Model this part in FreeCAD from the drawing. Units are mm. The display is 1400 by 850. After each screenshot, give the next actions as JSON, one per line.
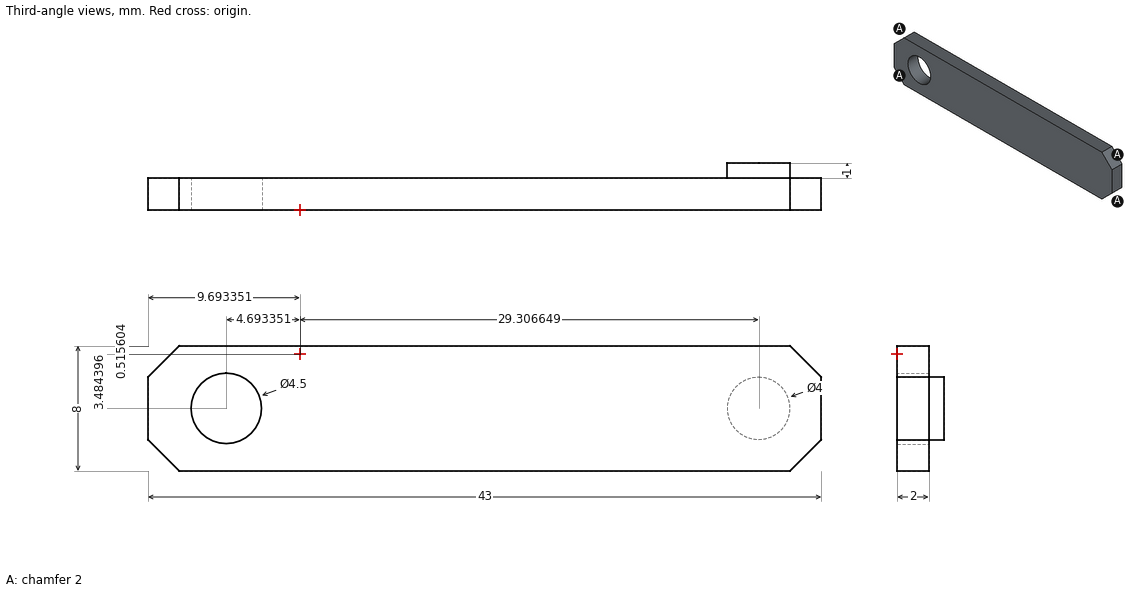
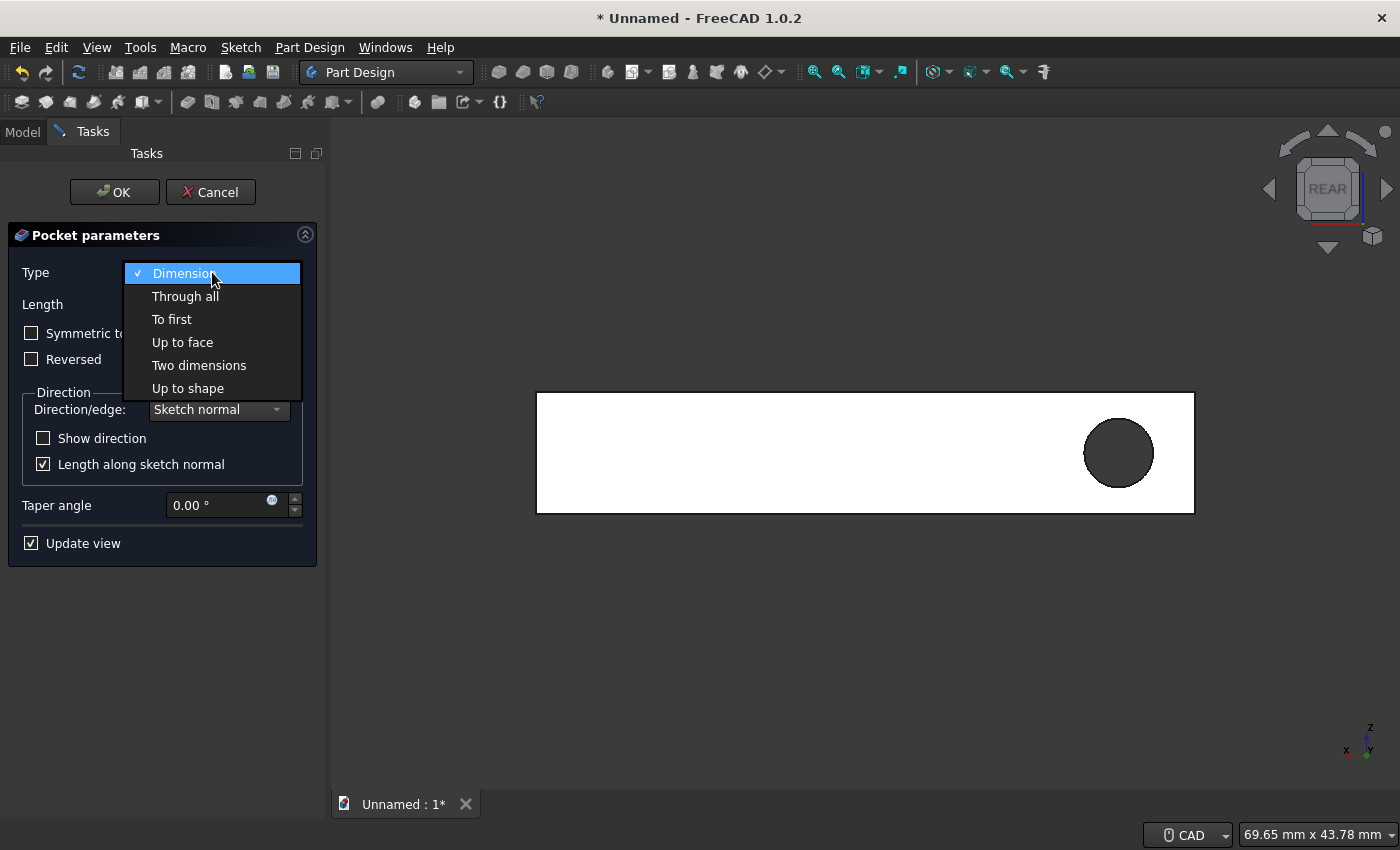
{"action": "left_click", "coordinate": [212, 296]}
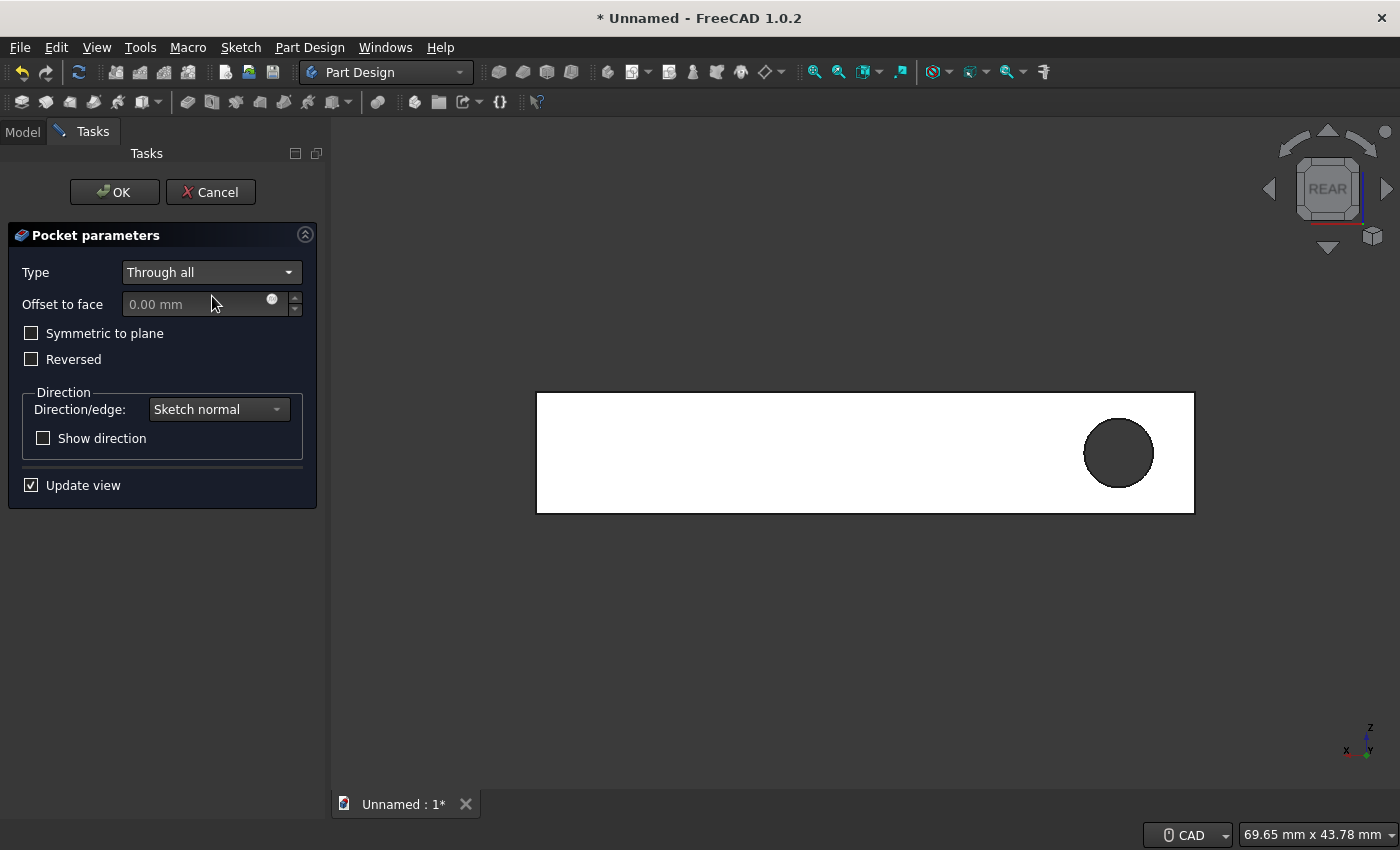
{"action": "left_click", "coordinate": [115, 192]}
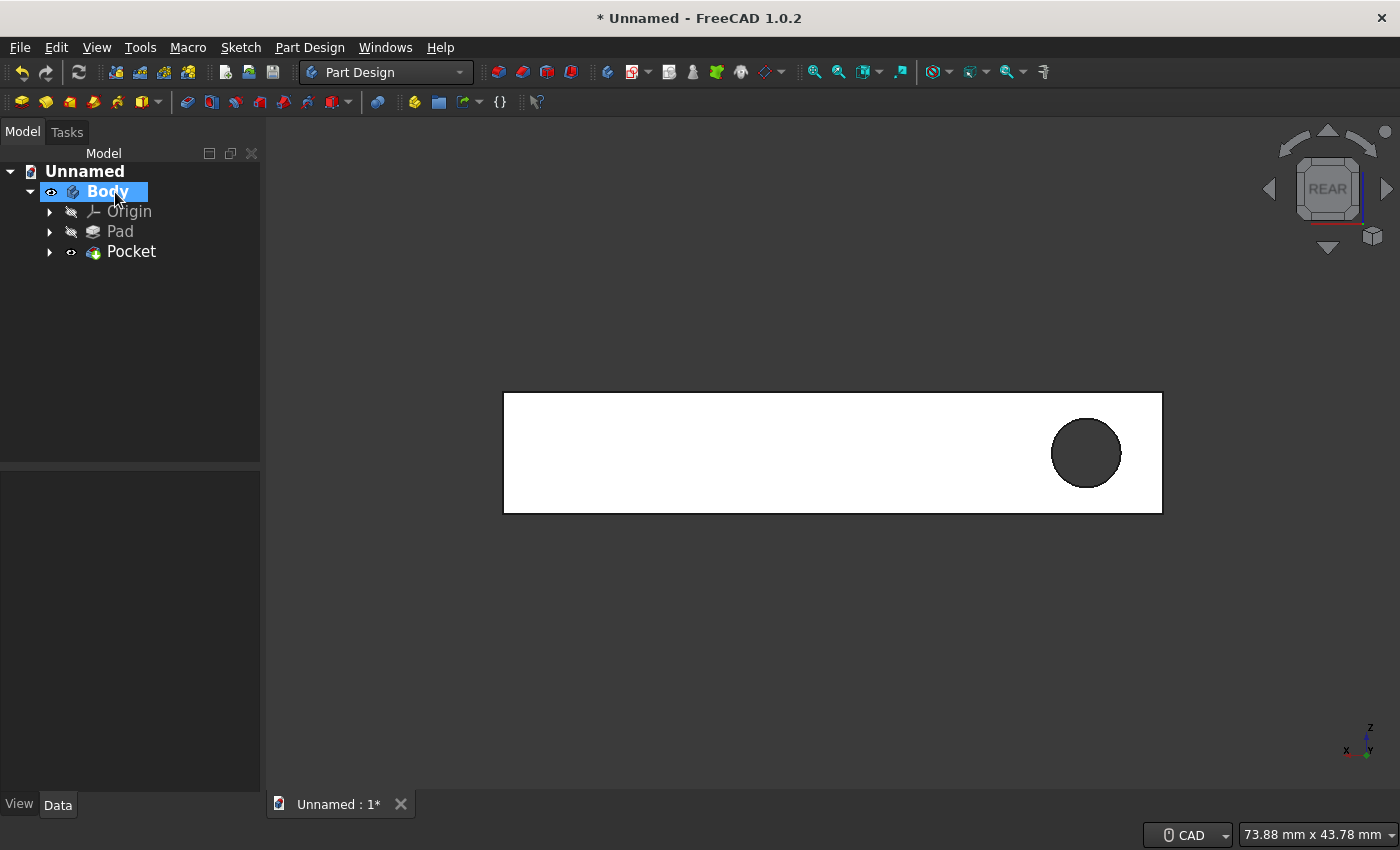
{"action": "left_click", "coordinate": [644, 452]}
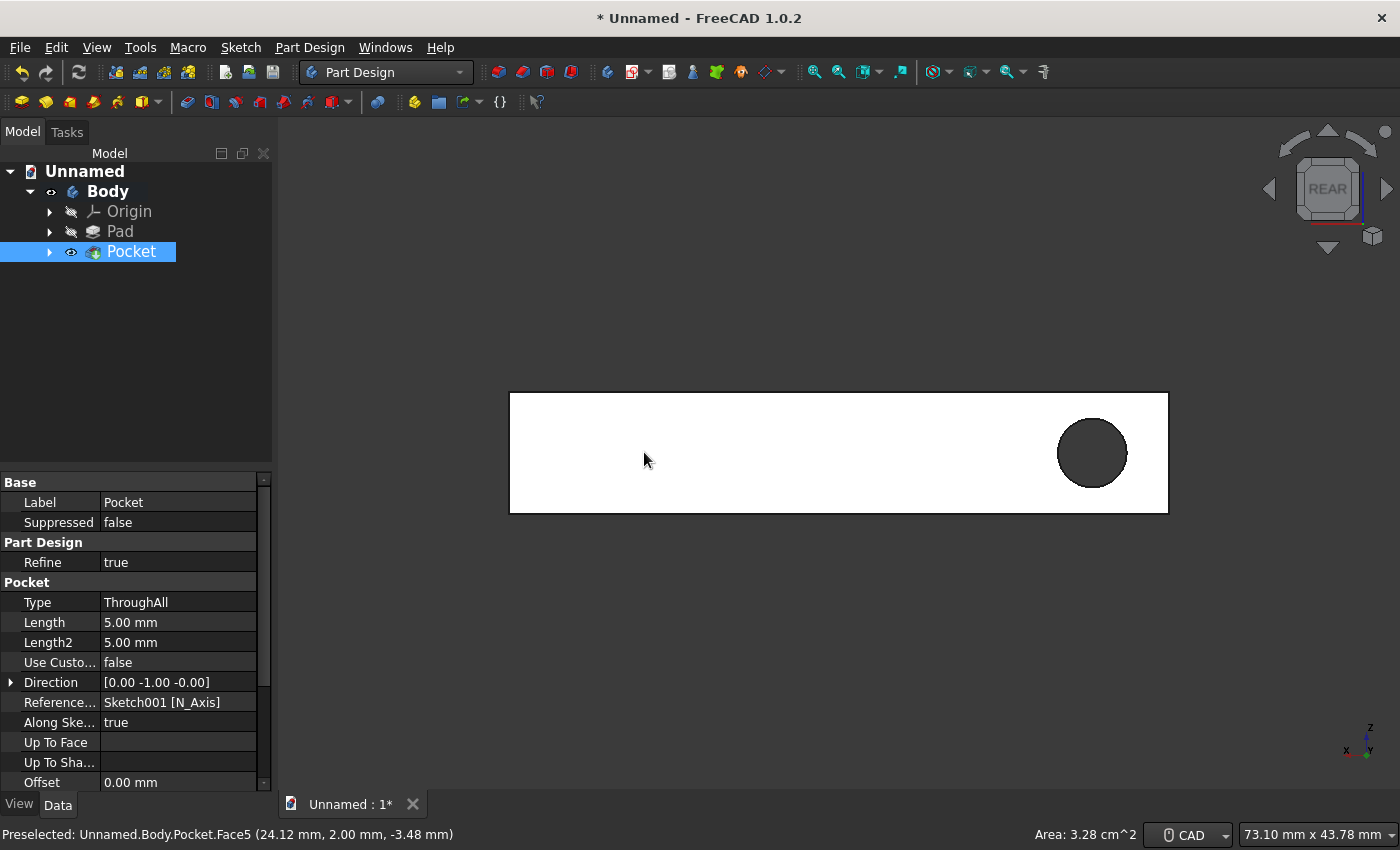
{"action": "left_click", "coordinate": [632, 72]}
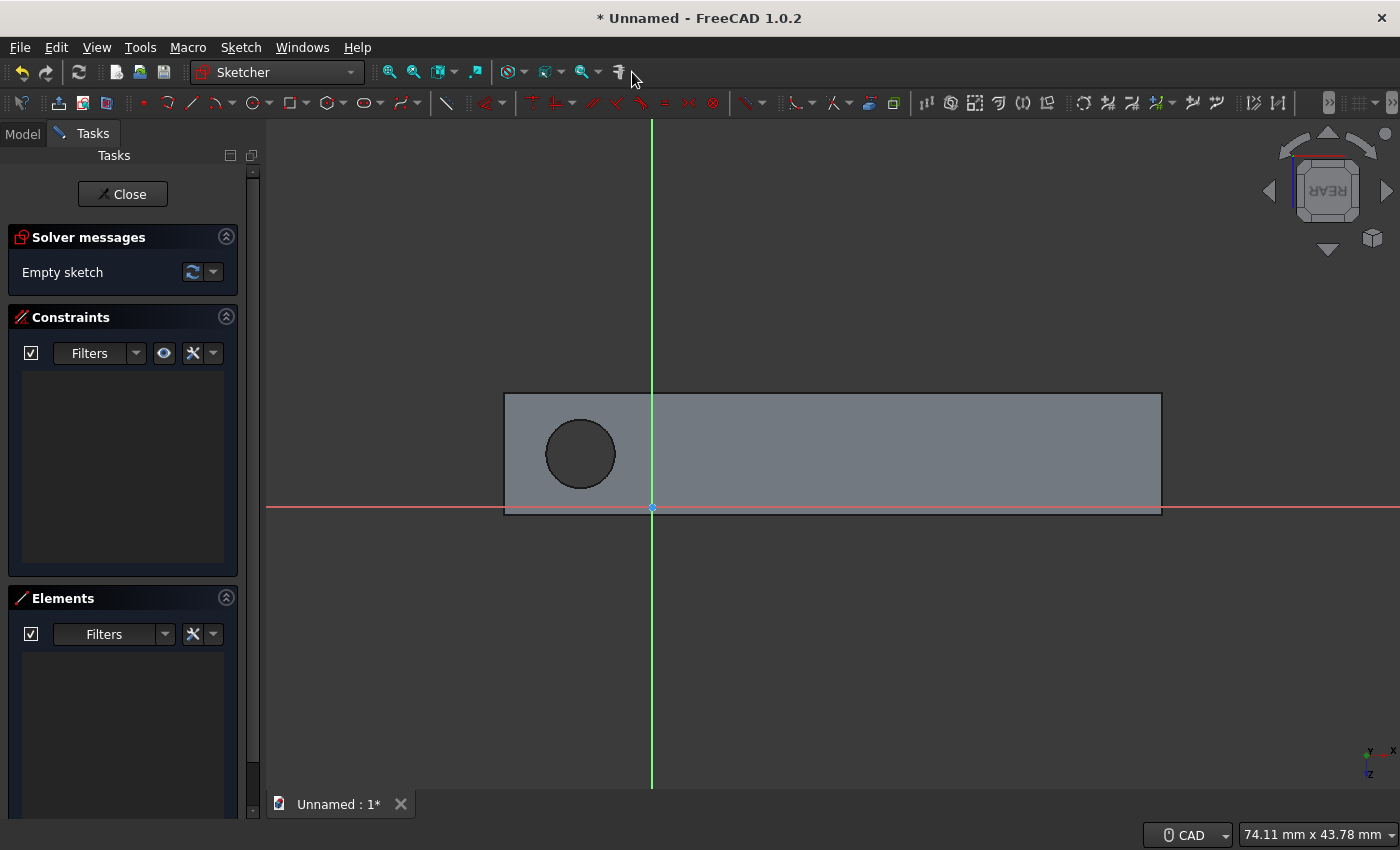
{"action": "scroll", "coordinate": [1153, 454], "scroll_direction": "up", "scroll_amount": 10}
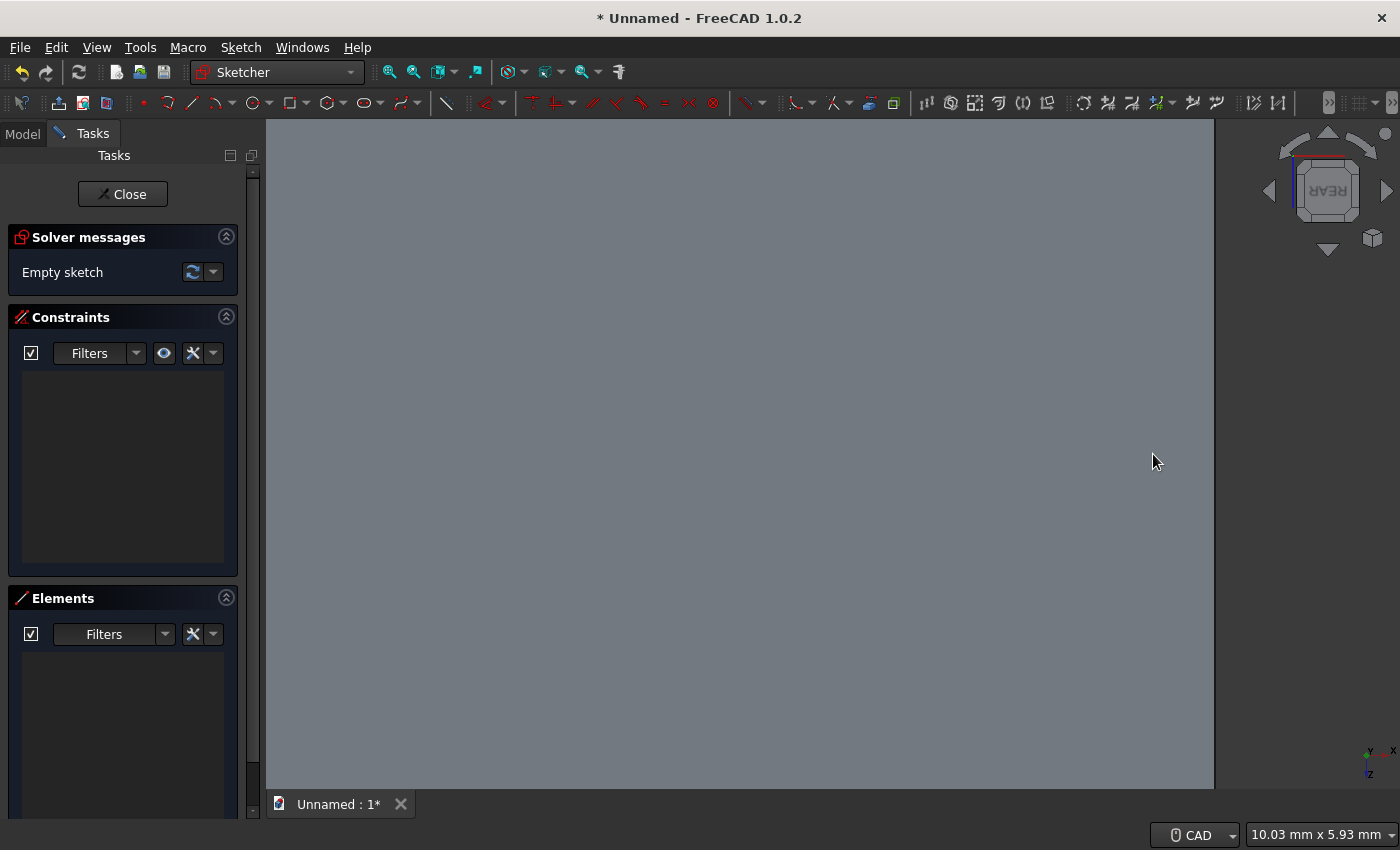
{"action": "left_click", "coordinate": [254, 104]}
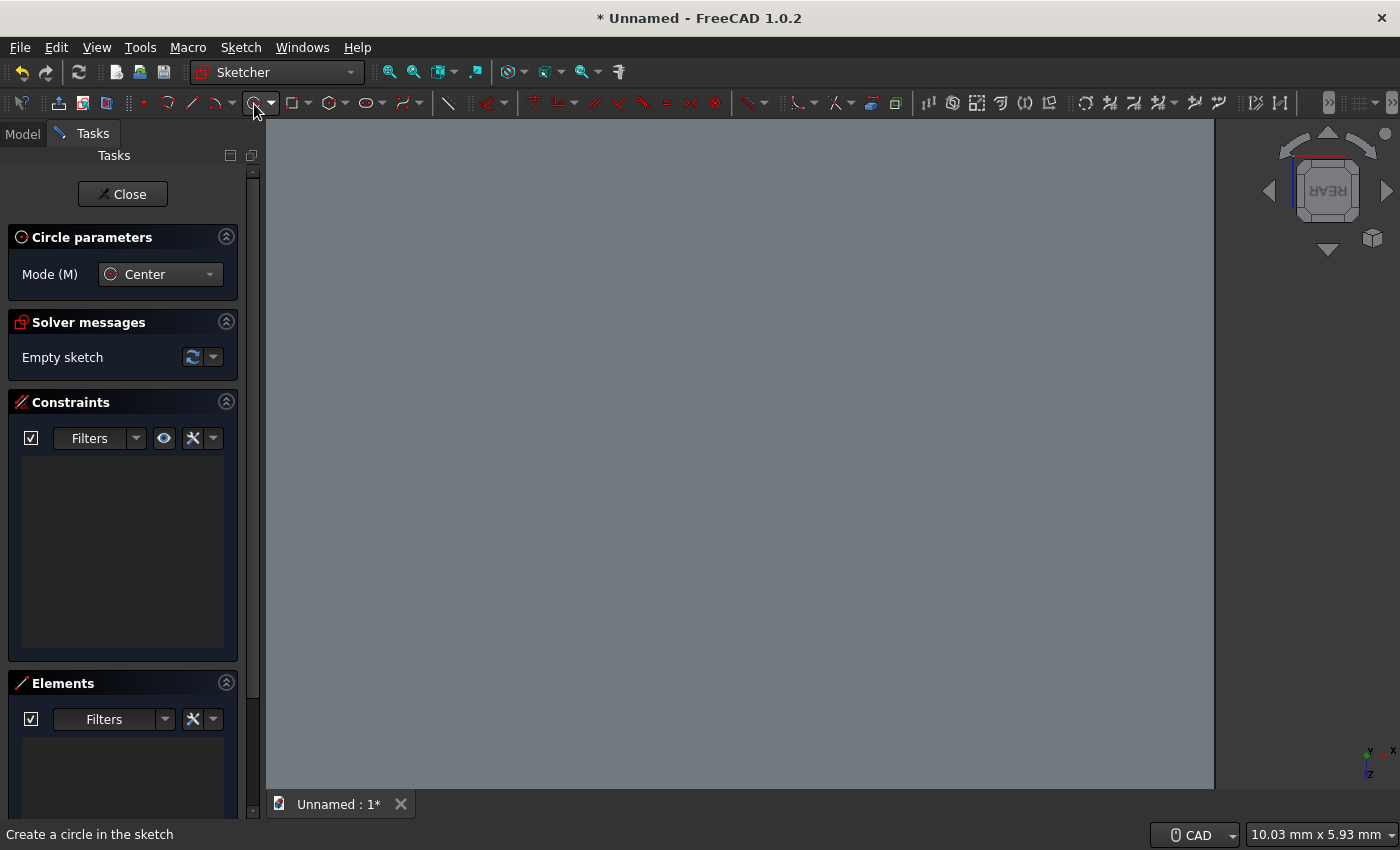
{"action": "left_click", "coordinate": [762, 451]}
{"action": "left_click", "coordinate": [922, 291]}
{"action": "key", "text": "Escape"}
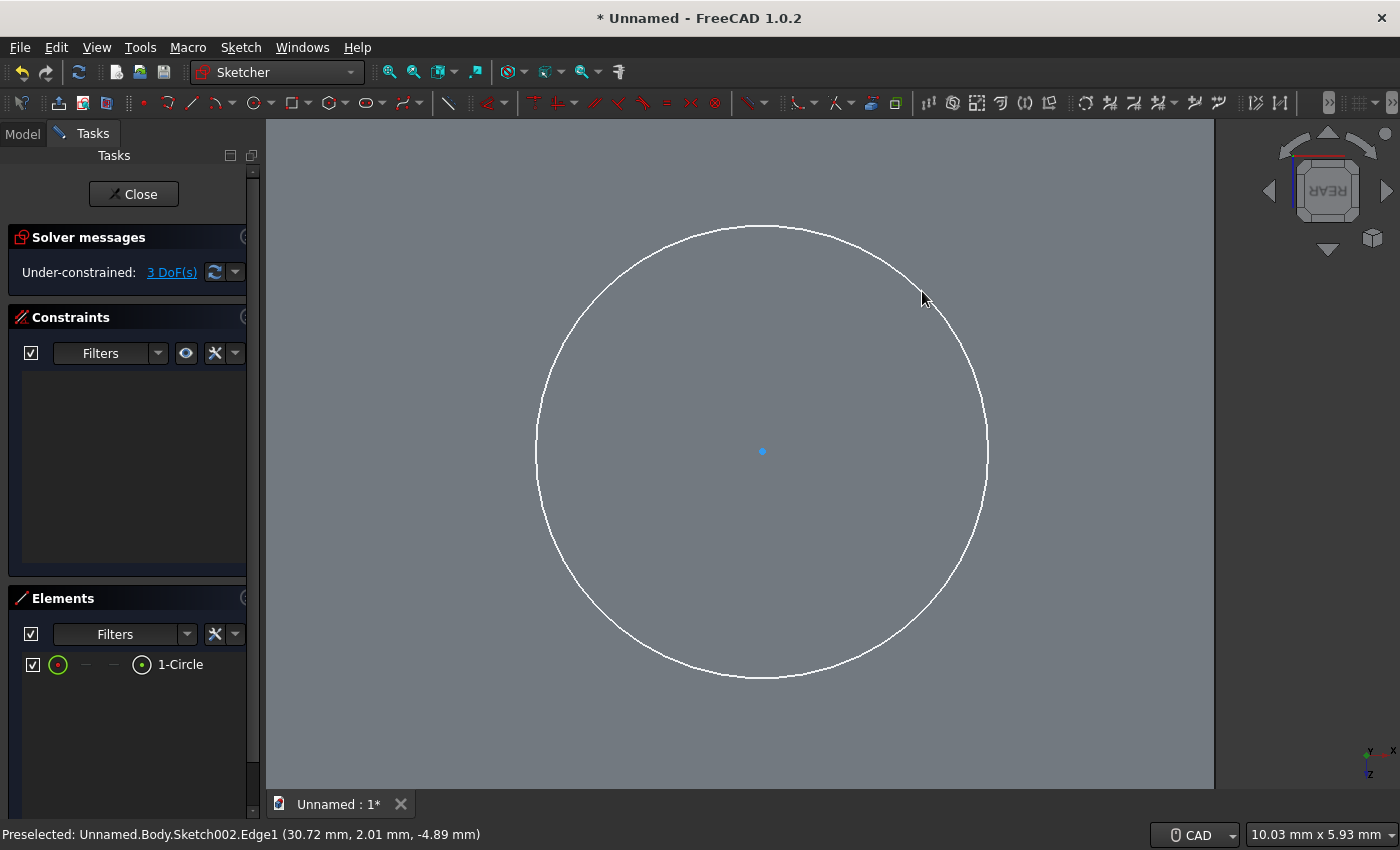
{"action": "left_click", "coordinate": [488, 104]}